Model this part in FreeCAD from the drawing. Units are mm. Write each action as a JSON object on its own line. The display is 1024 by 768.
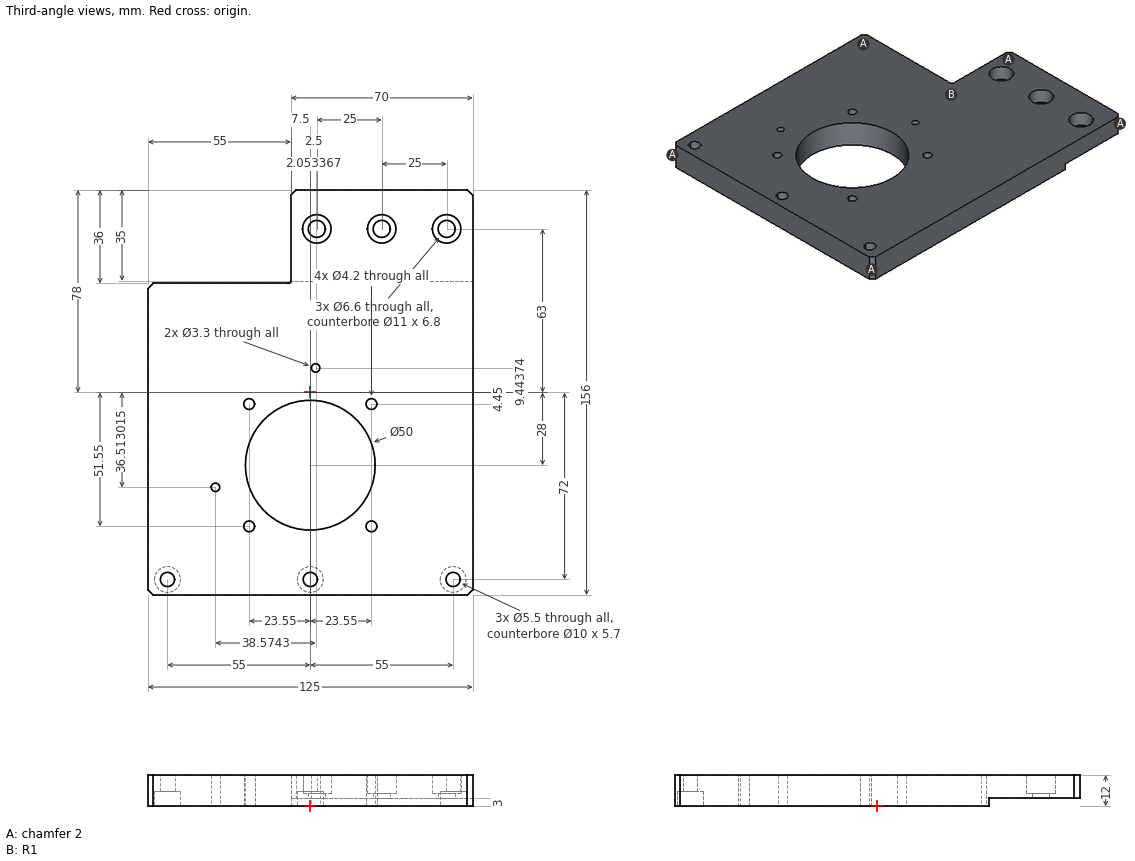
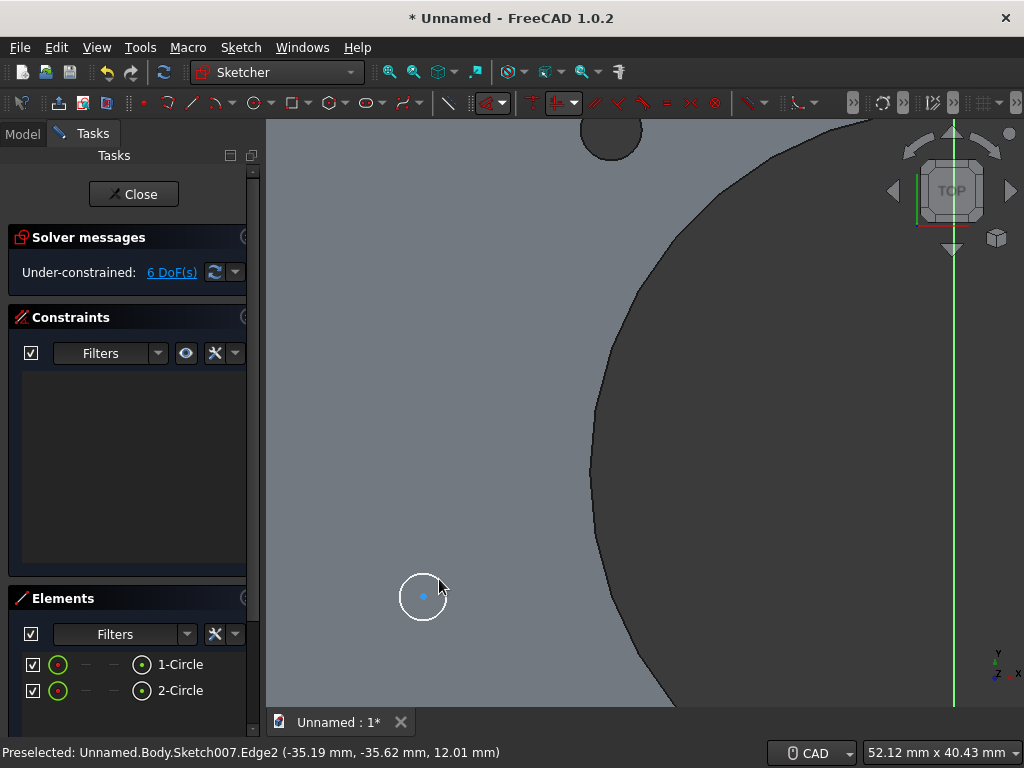
{"action": "scroll", "coordinate": [423, 597], "scroll_direction": "down", "scroll_amount": 3}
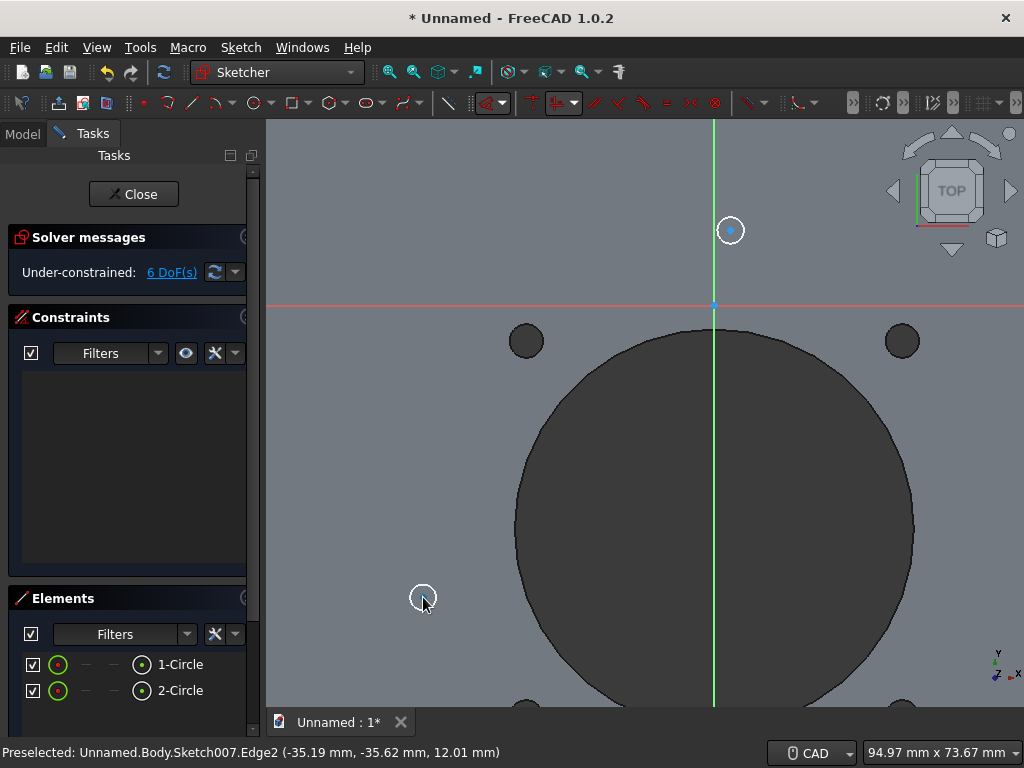
{"action": "left_click", "coordinate": [740, 221]}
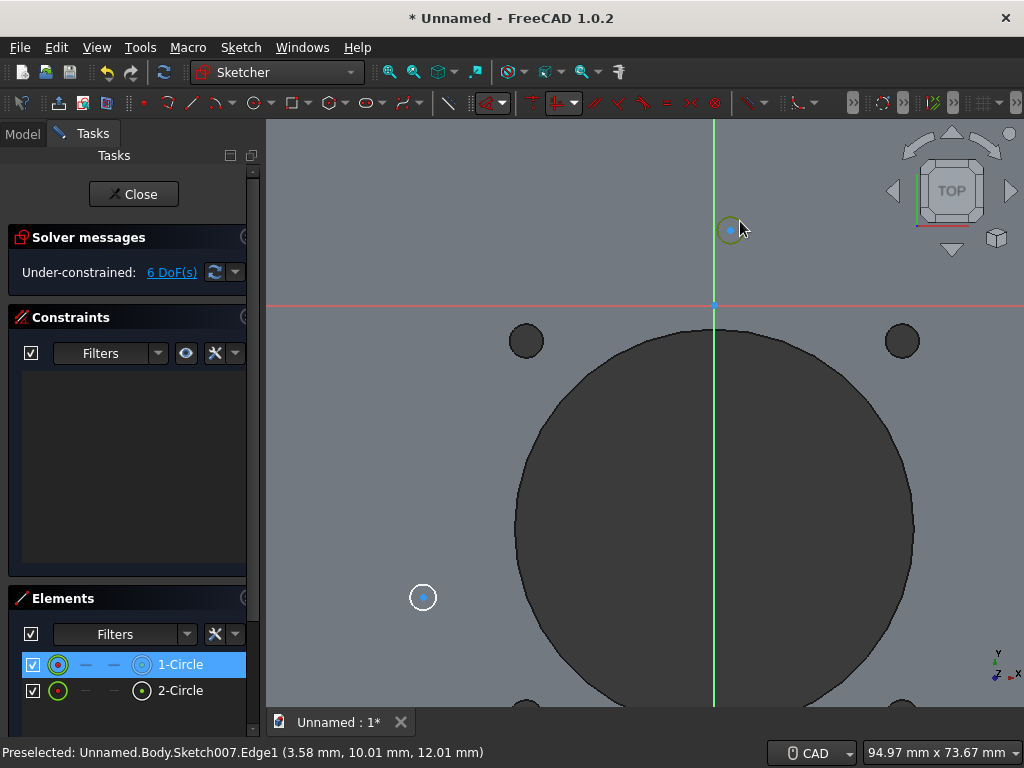
{"action": "left_click", "coordinate": [432, 588]}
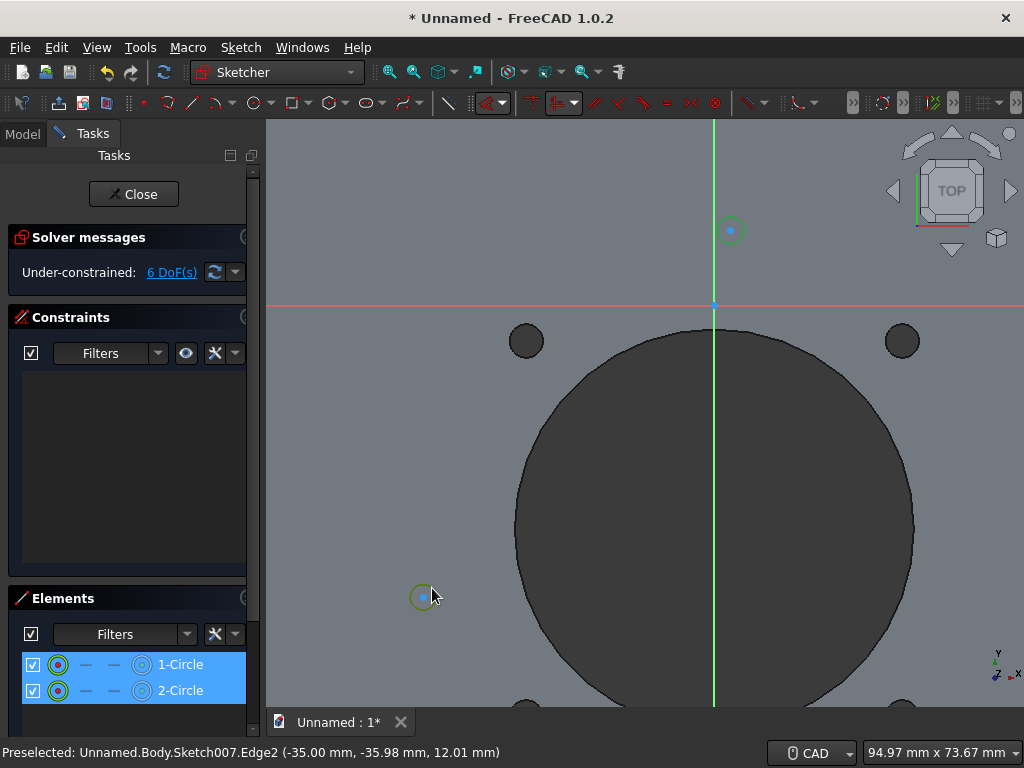
{"action": "left_click", "coordinate": [668, 104]}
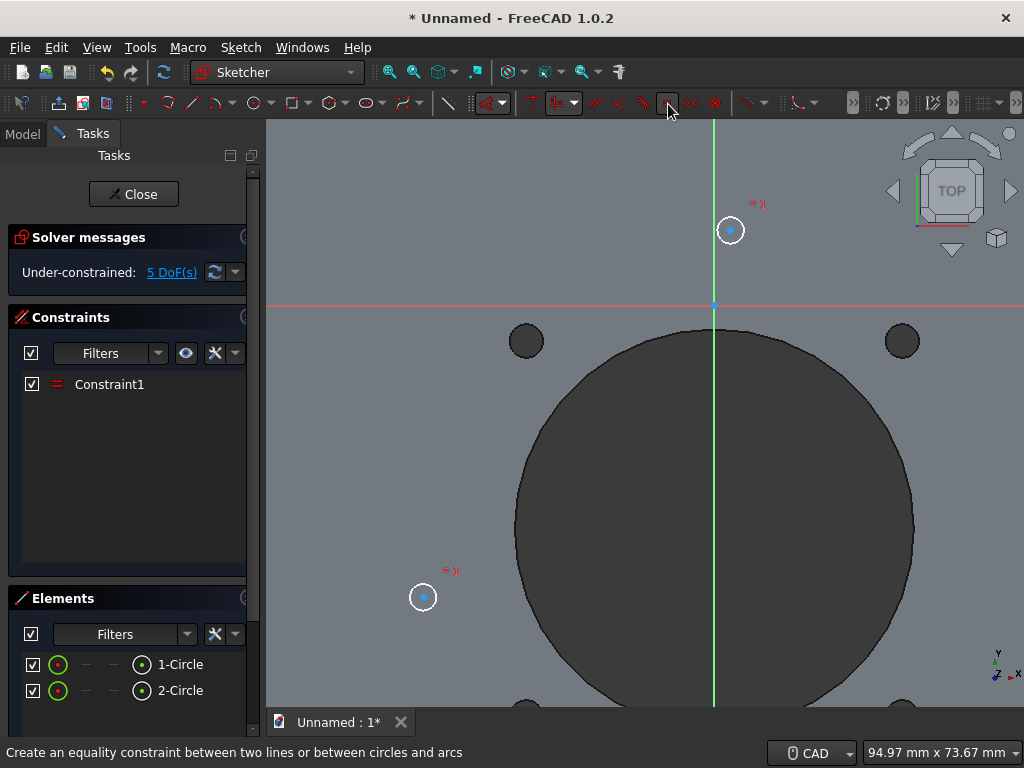
{"action": "scroll", "coordinate": [740, 221], "scroll_direction": "up", "scroll_amount": 3}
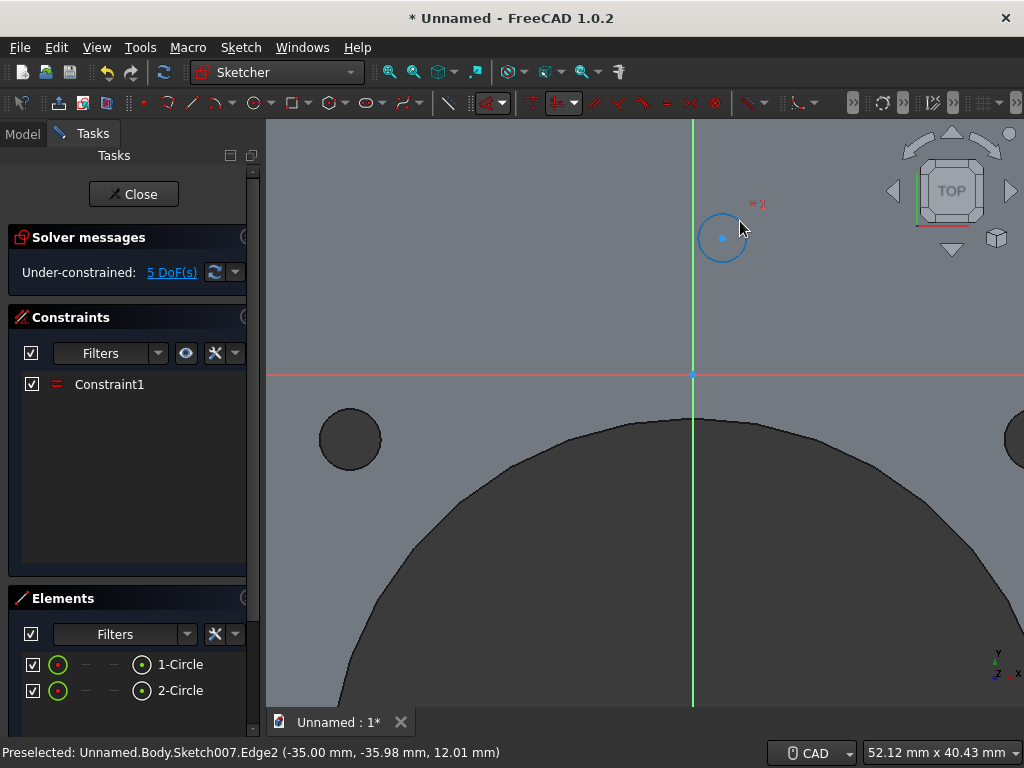
{"action": "left_click", "coordinate": [739, 221]}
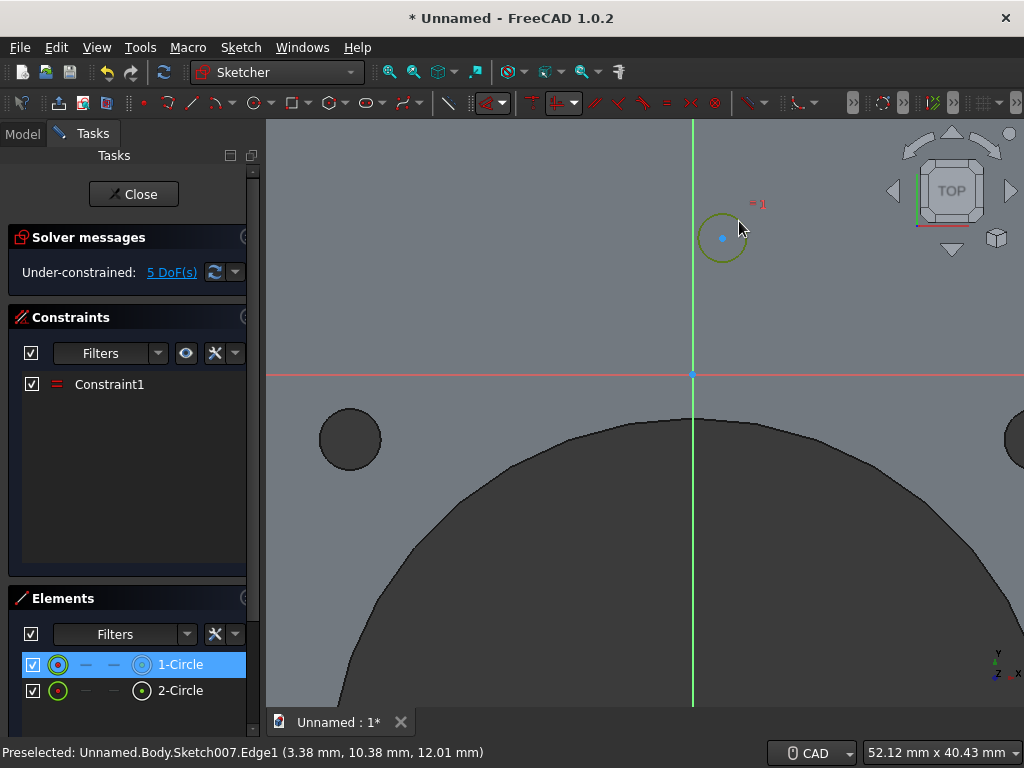
{"action": "left_click", "coordinate": [504, 104]}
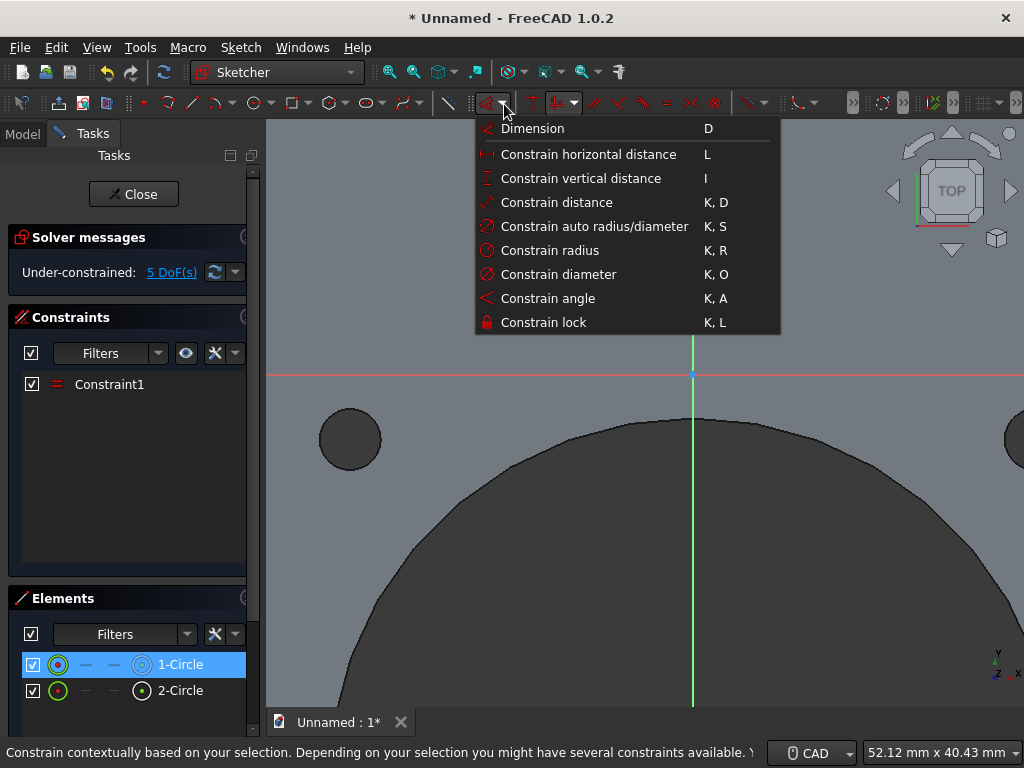
{"action": "left_click", "coordinate": [628, 274]}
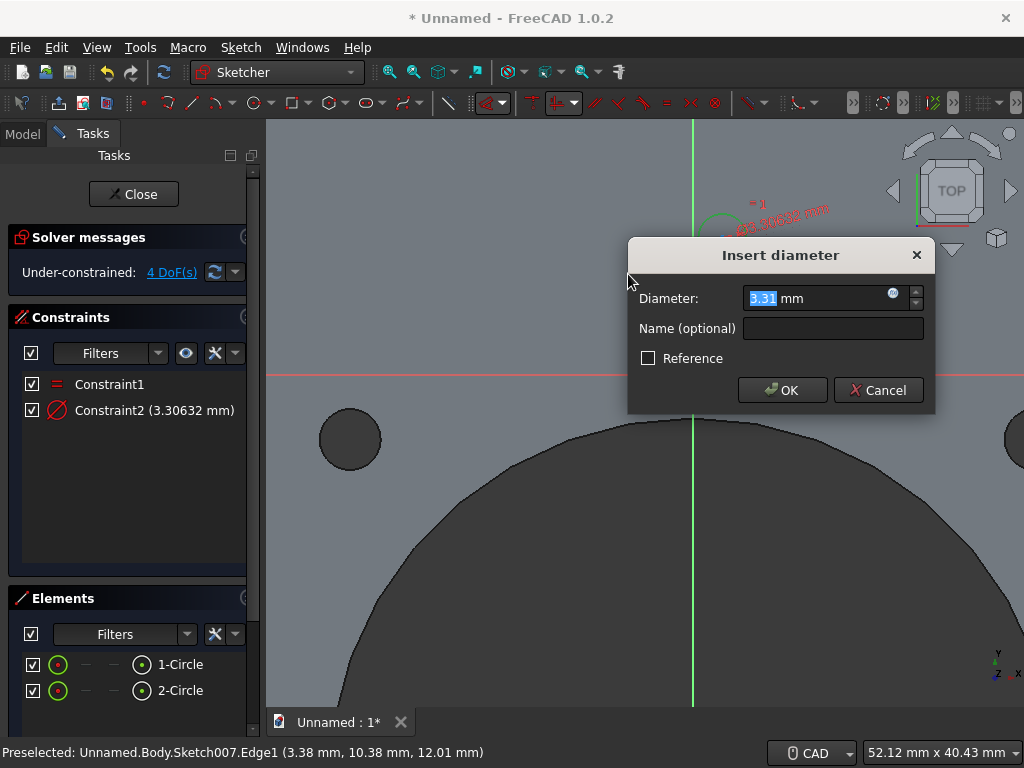
{"action": "type", "text": "3.3"}
{"action": "key", "text": "Return"}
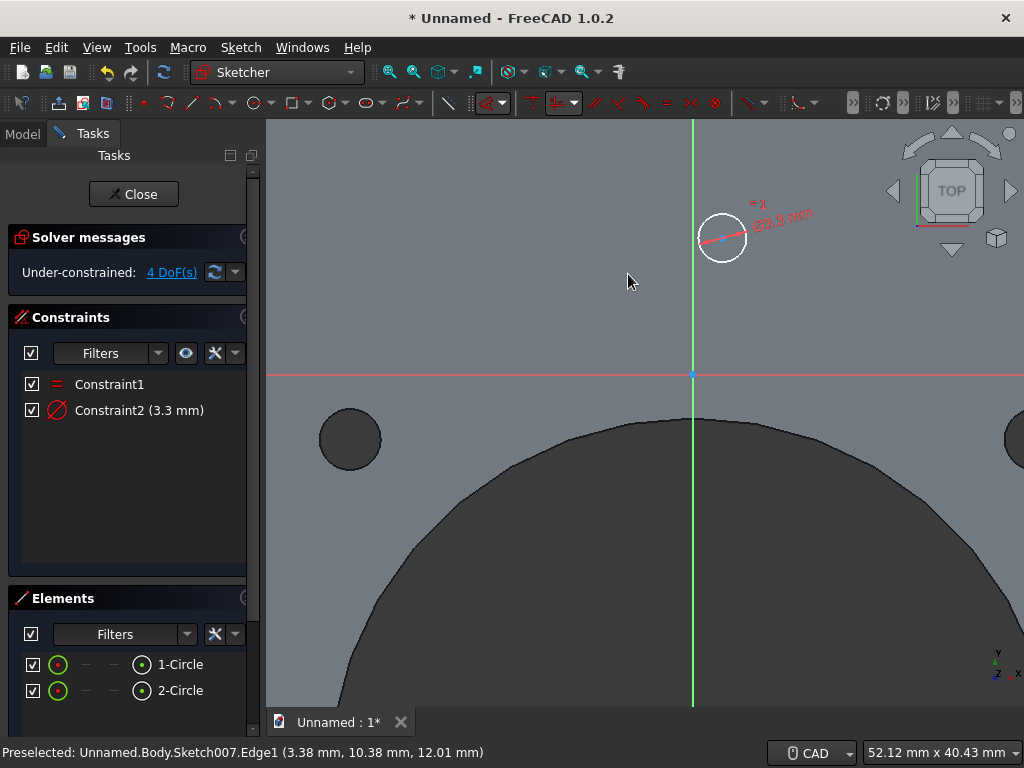
{"action": "left_click", "coordinate": [722, 238]}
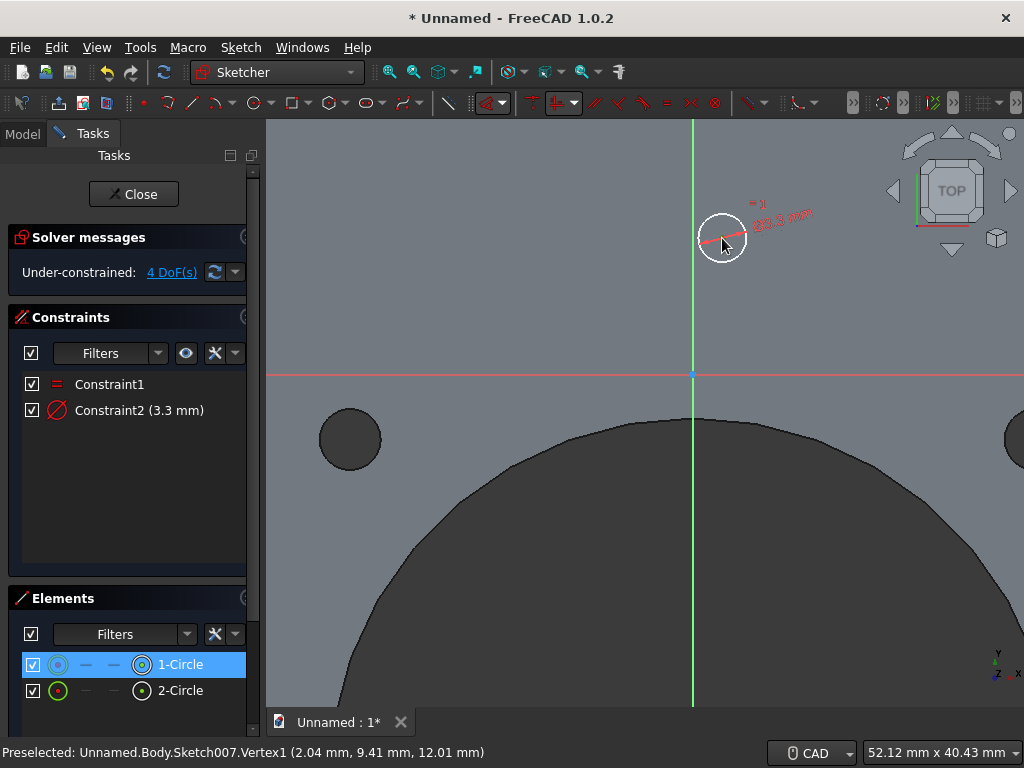
{"action": "left_click", "coordinate": [504, 104]}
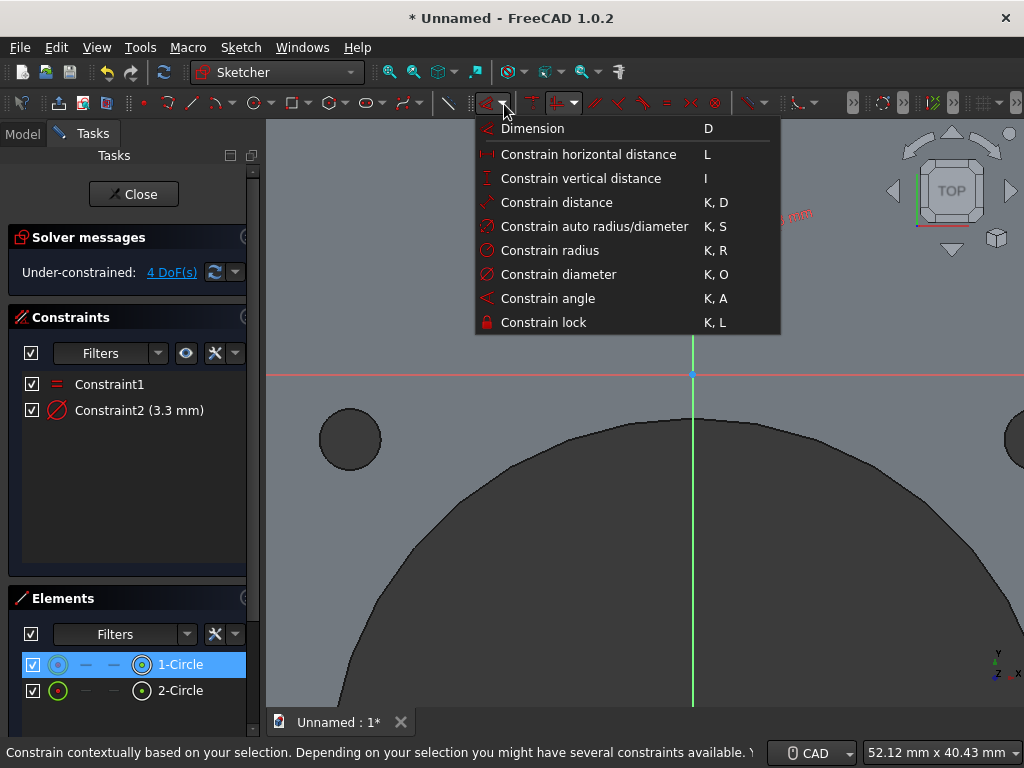
{"action": "left_click", "coordinate": [628, 178]}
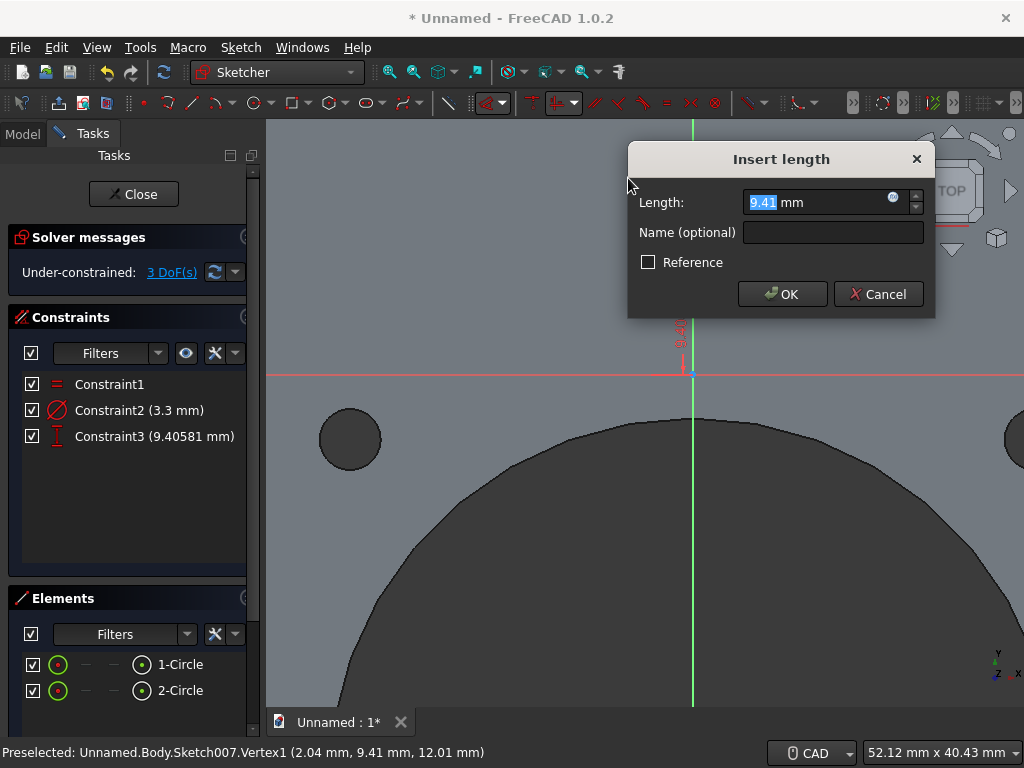
{"action": "type", "text": "9.44374"}
{"action": "key", "text": "Return"}